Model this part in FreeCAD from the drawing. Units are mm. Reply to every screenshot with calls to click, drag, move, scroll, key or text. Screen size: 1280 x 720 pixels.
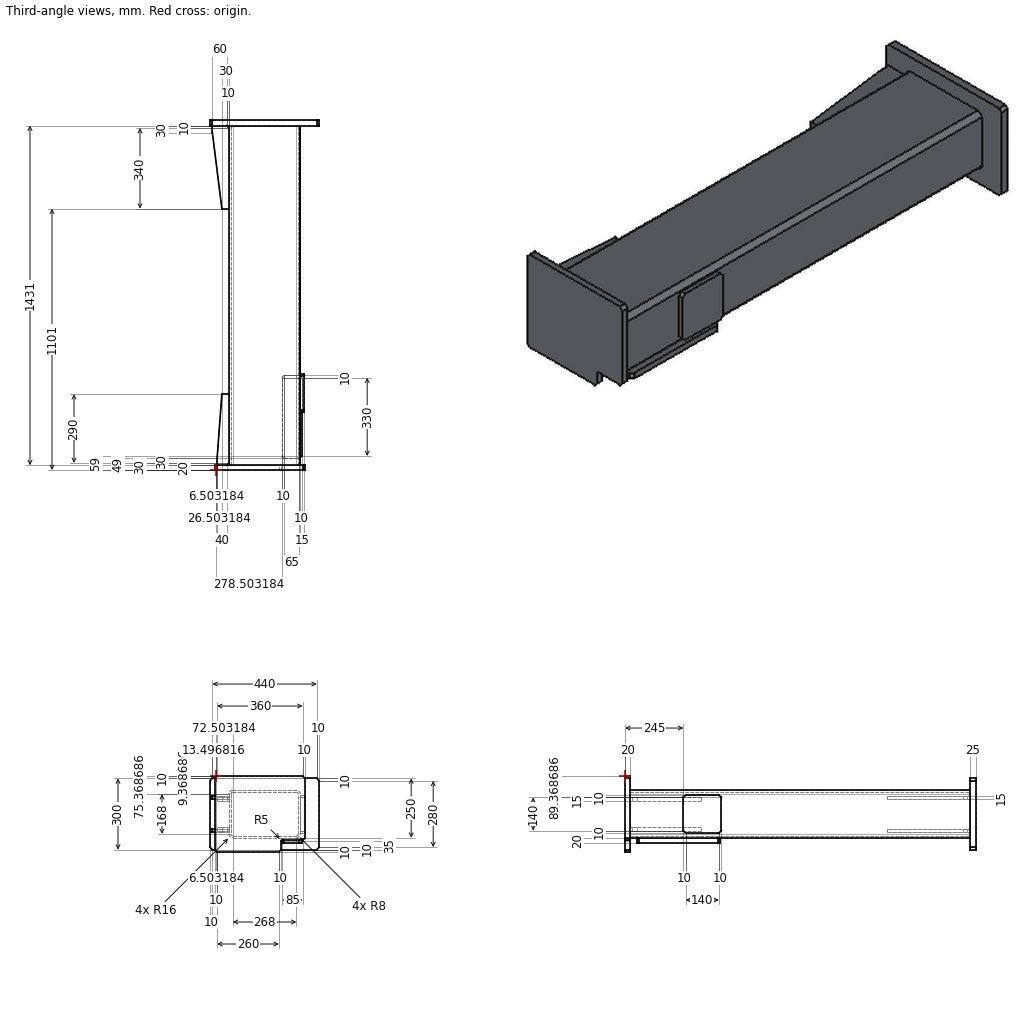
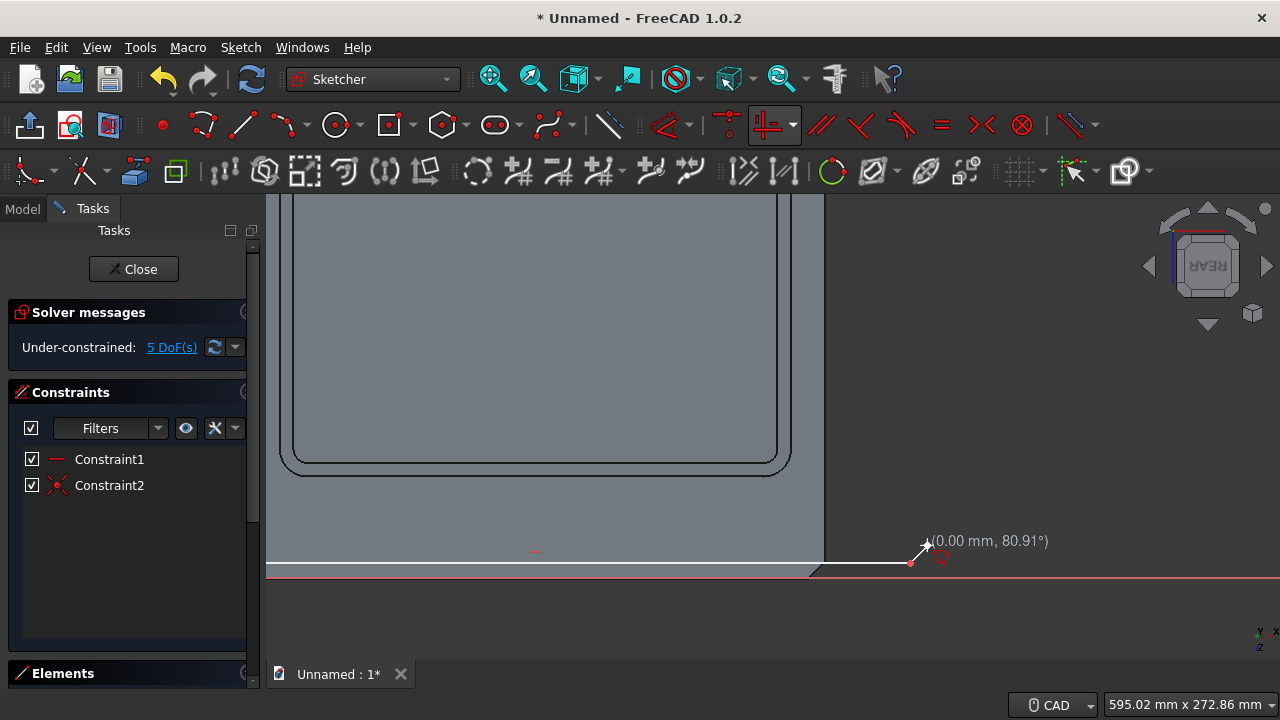
scroll(910, 563, down, 3)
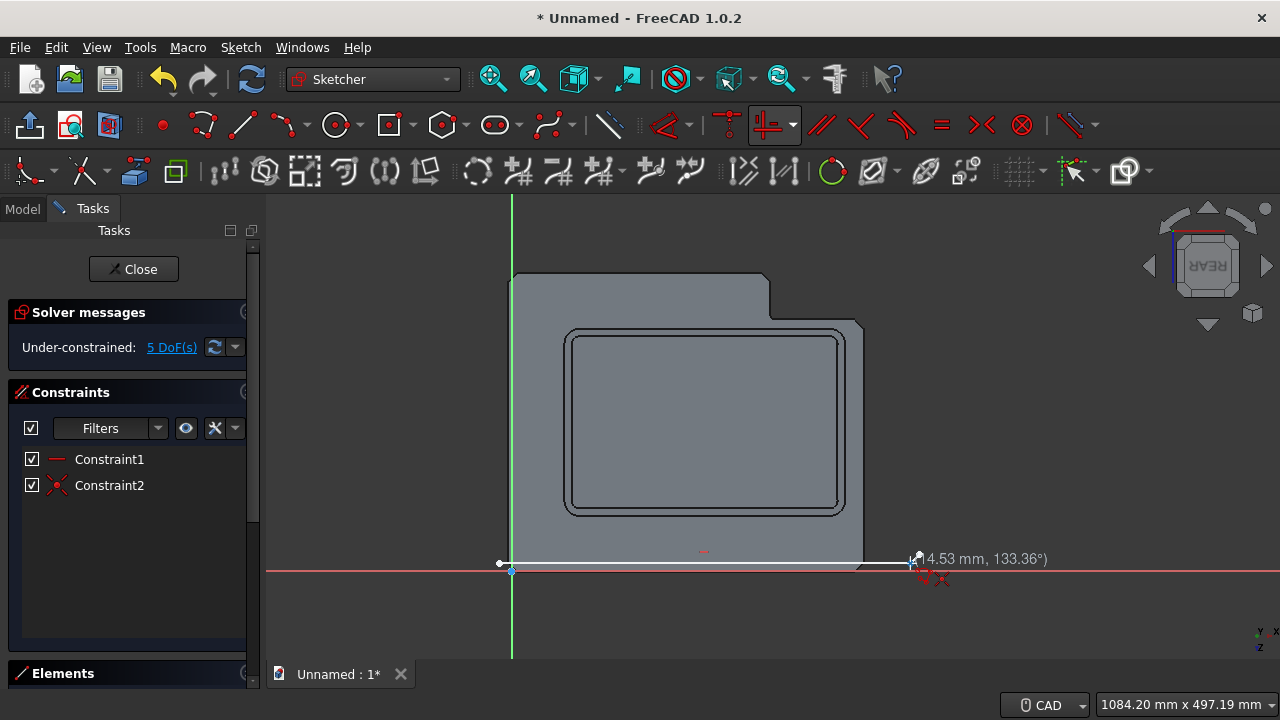
click(920, 291)
click(910, 282)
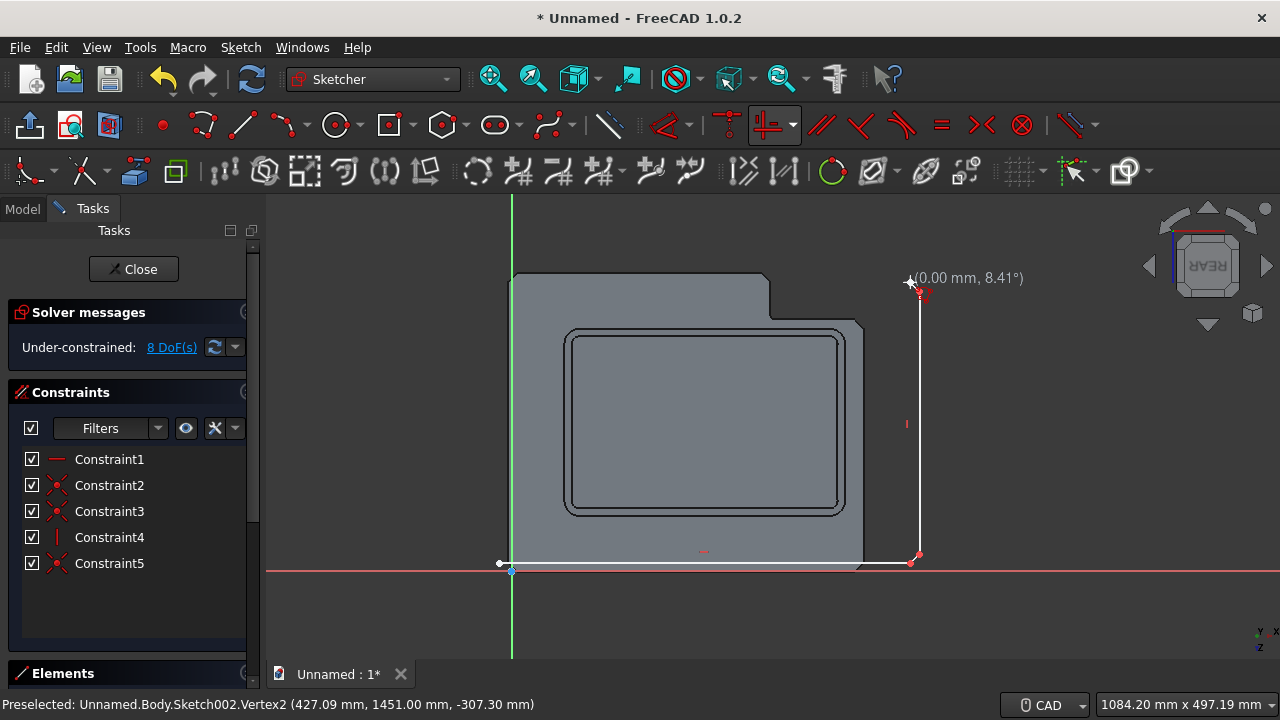
scroll(499, 282, up, 2)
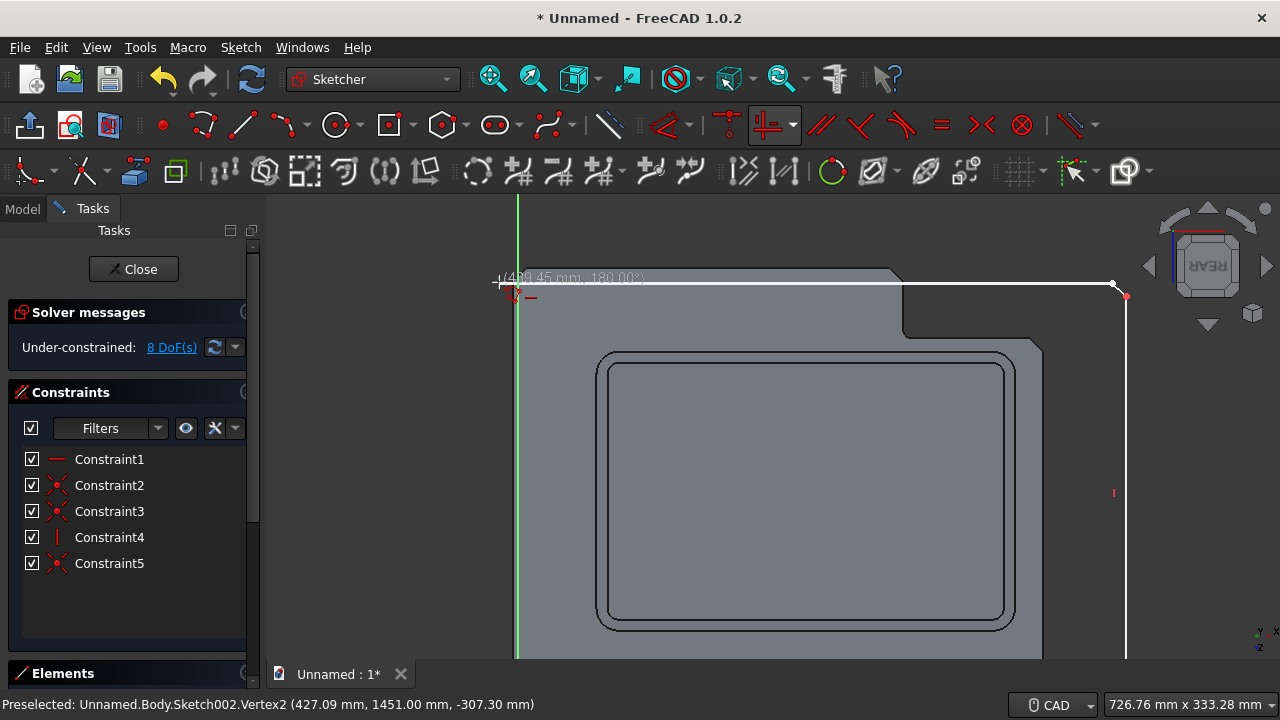
click(499, 282)
click(485, 296)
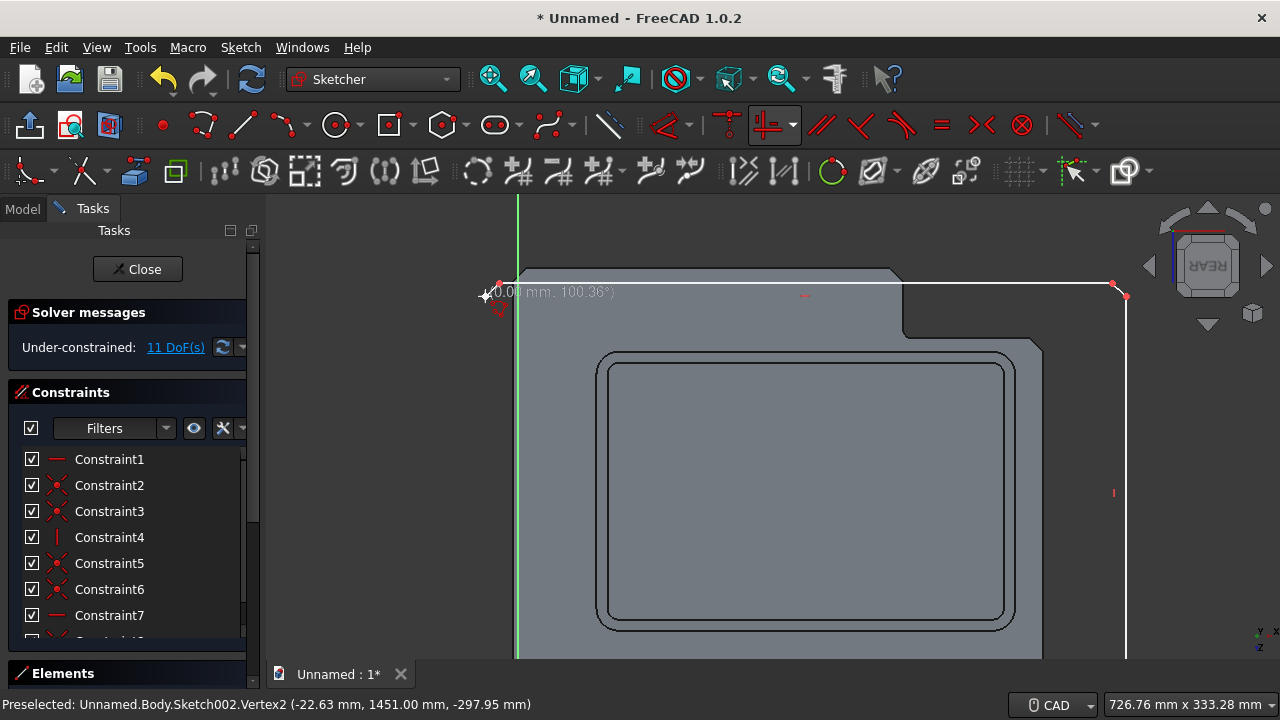
scroll(499, 281, down, 2)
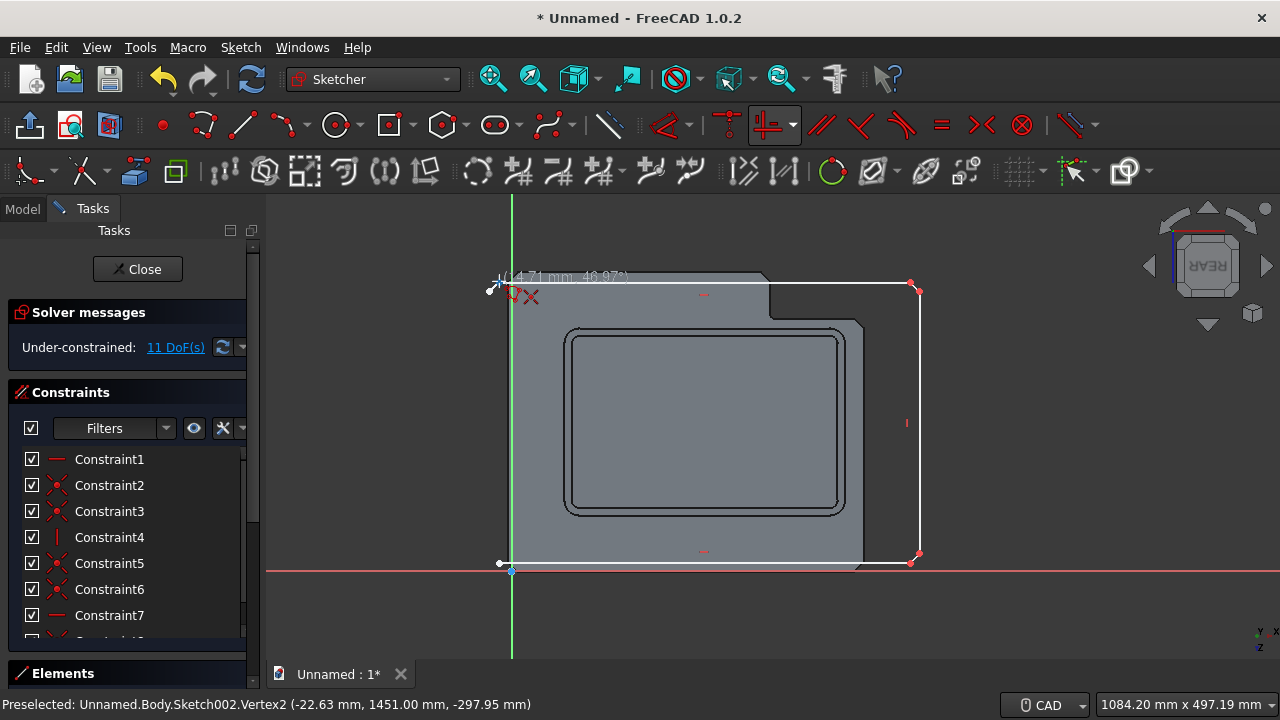
click(490, 553)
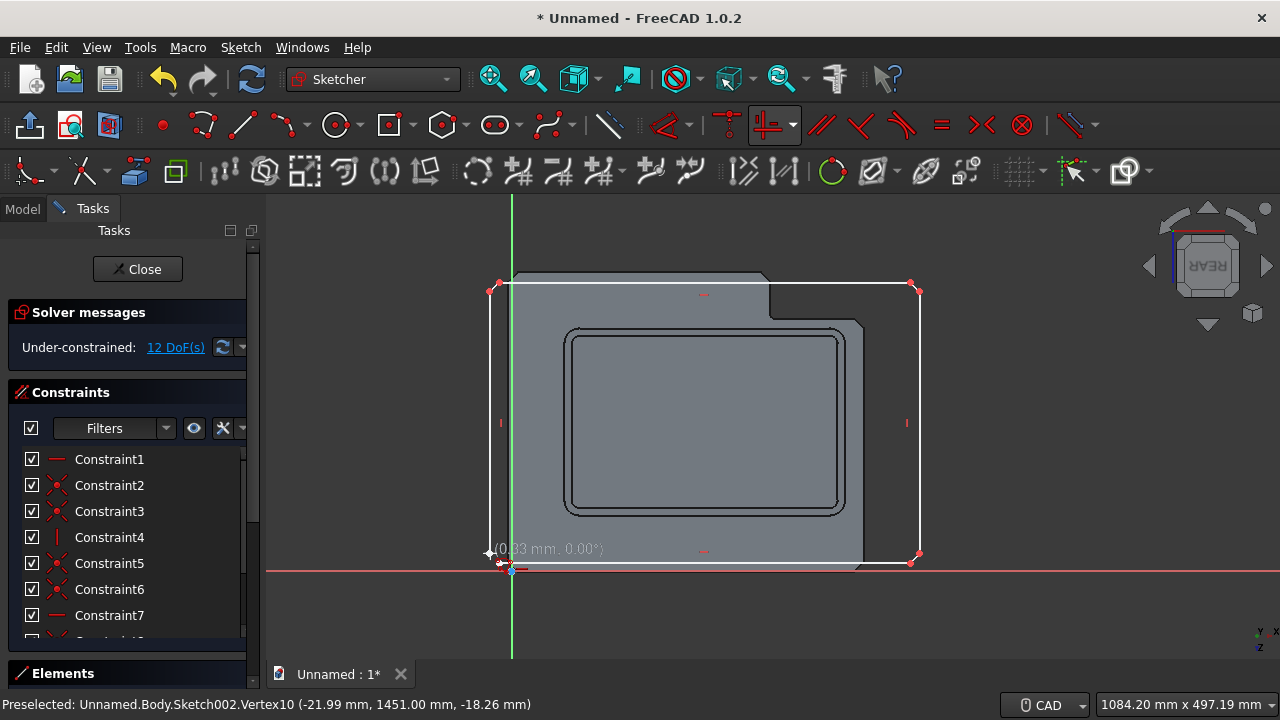
scroll(499, 562, up, 3)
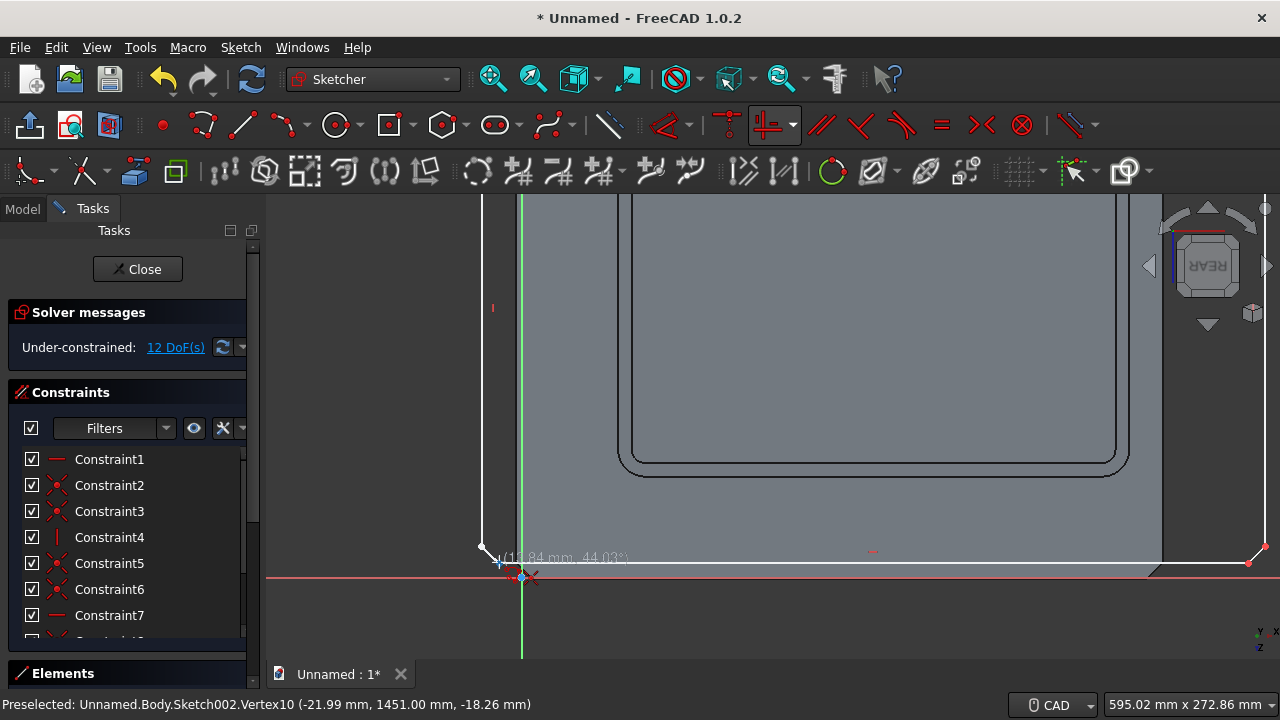
click(499, 563)
key(Escape)
key(Escape)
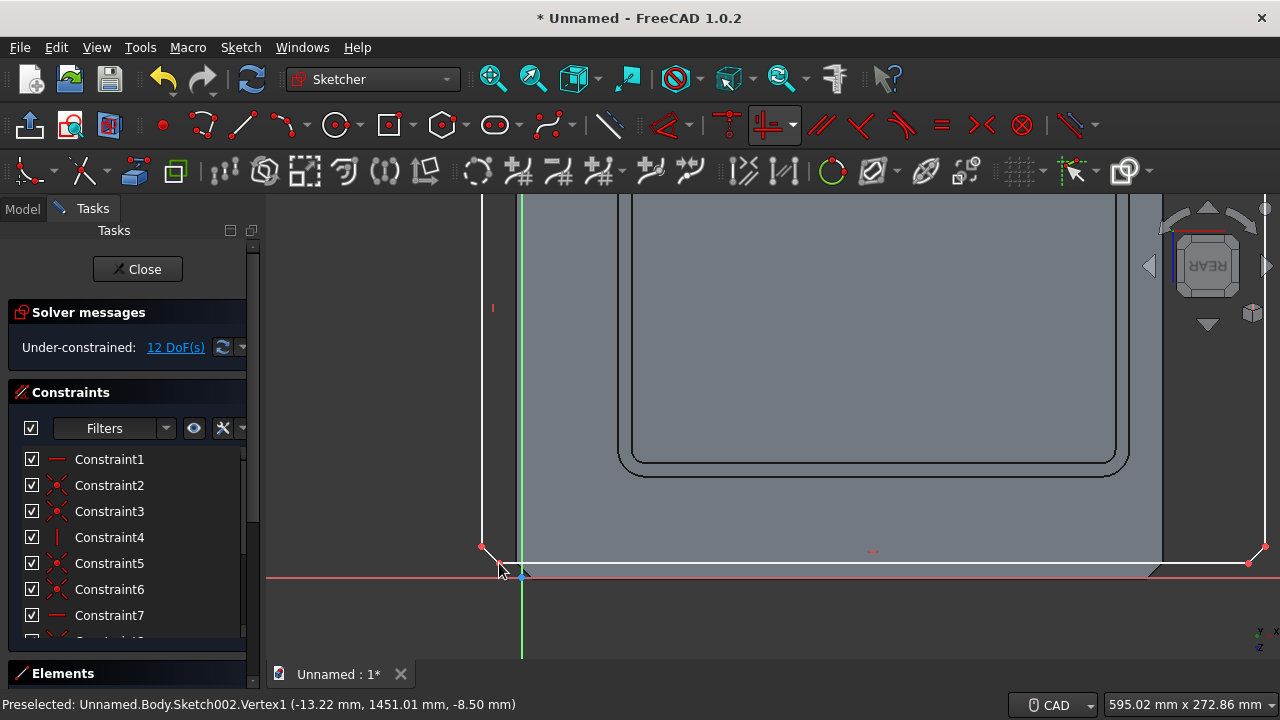
click(664, 126)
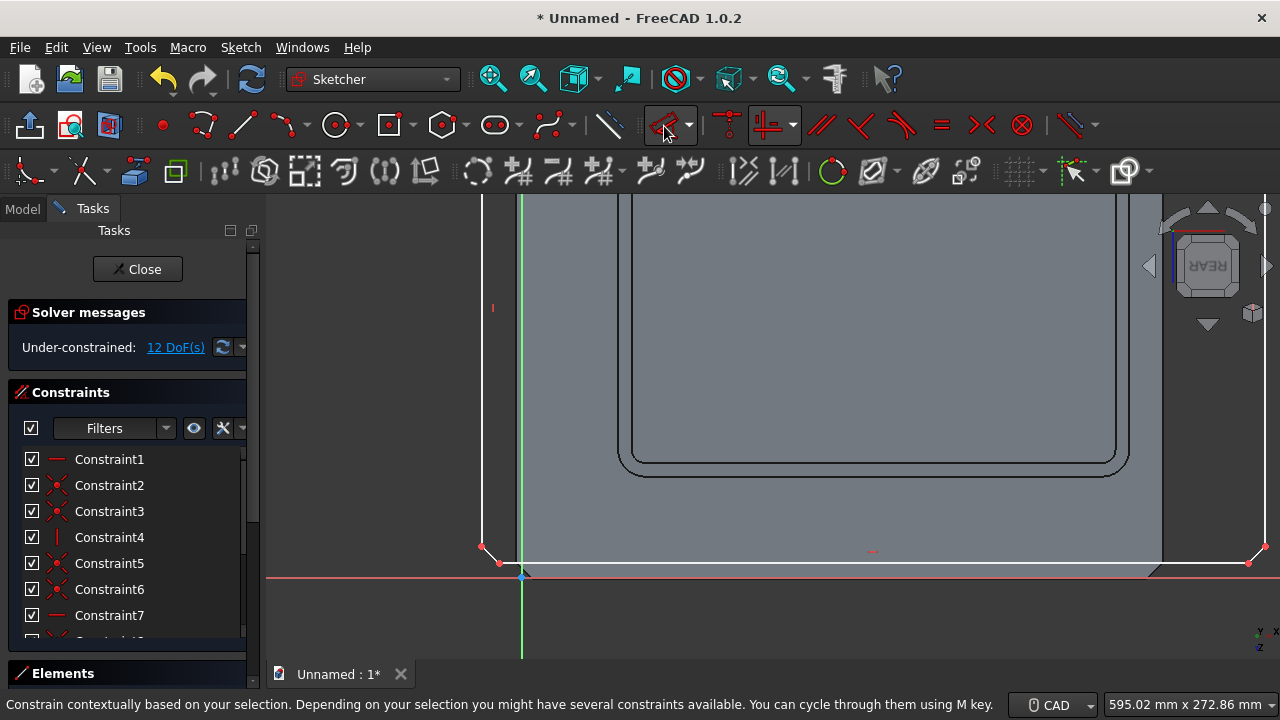
click(724, 563)
click(807, 597)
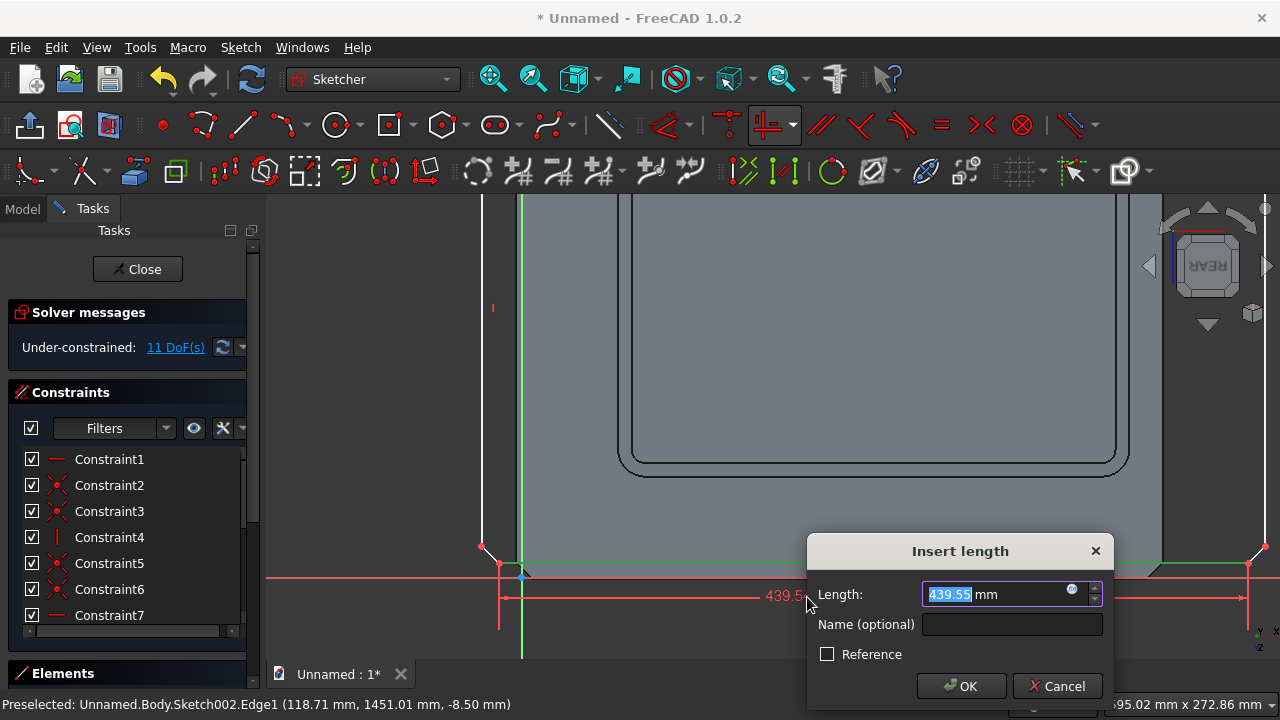
text(440)
key(Return)